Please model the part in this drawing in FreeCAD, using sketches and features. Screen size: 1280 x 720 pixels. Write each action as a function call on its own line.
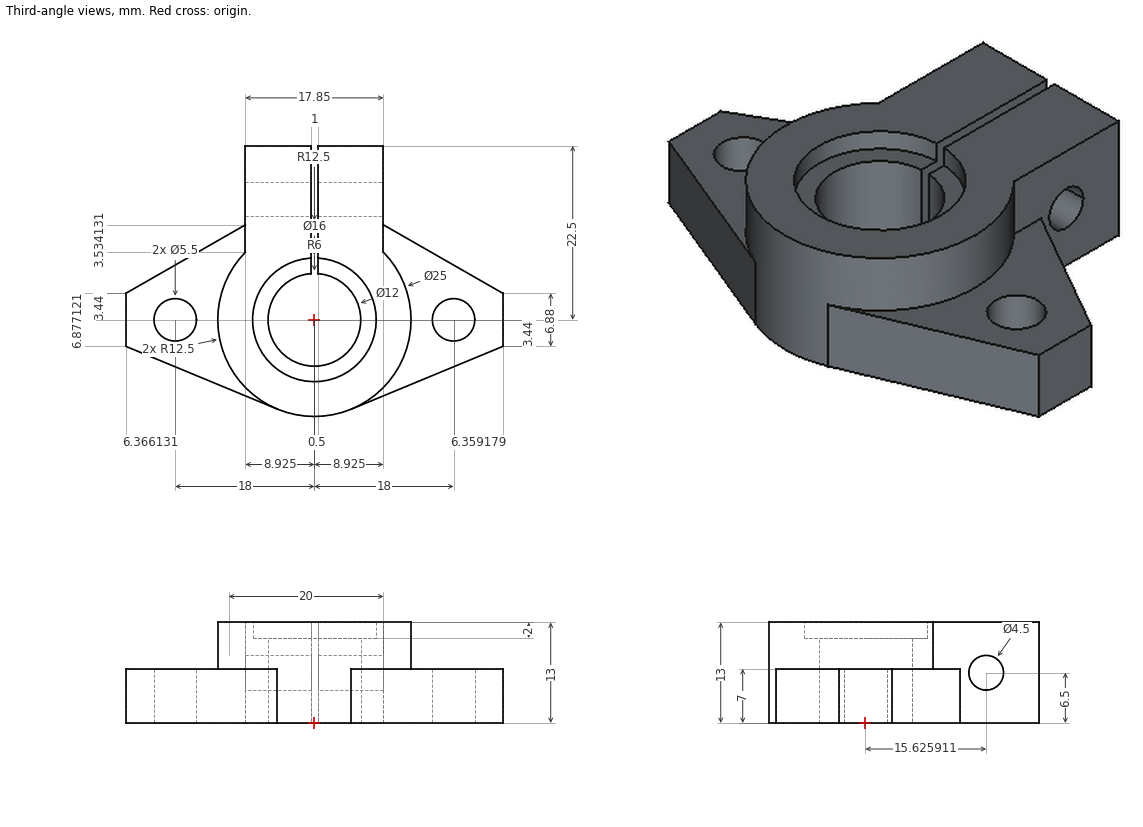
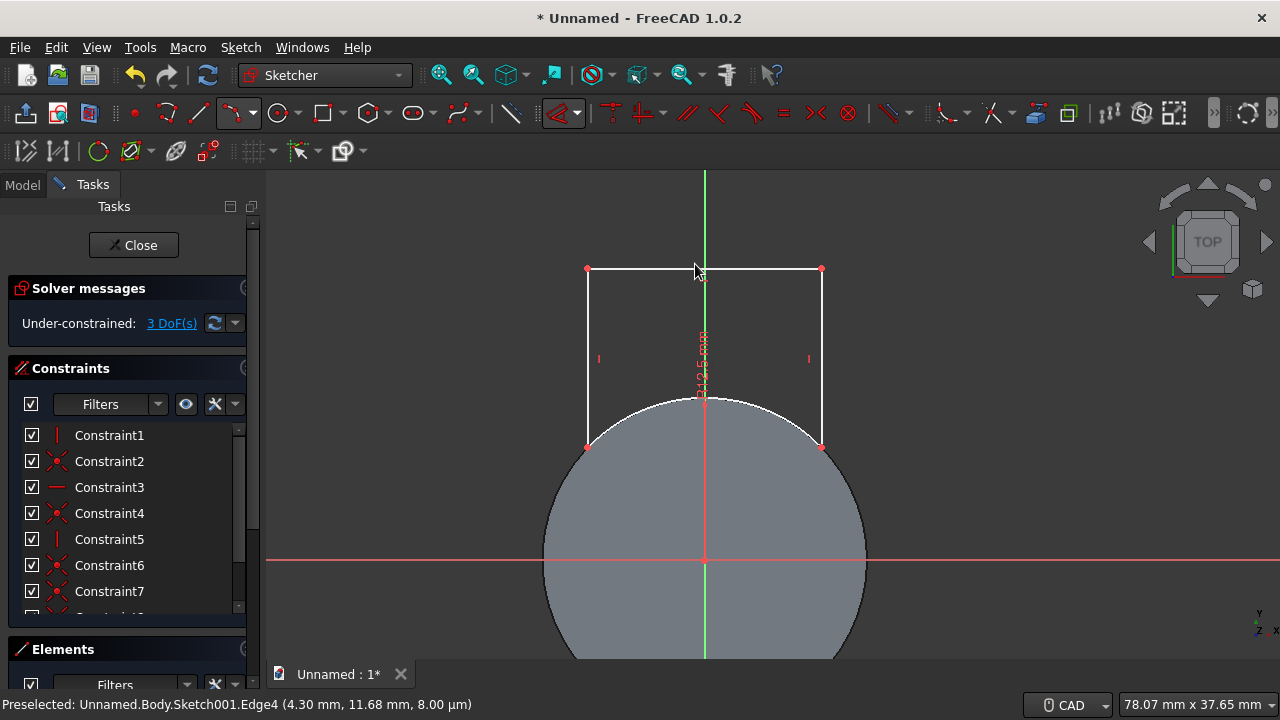
click(752, 269)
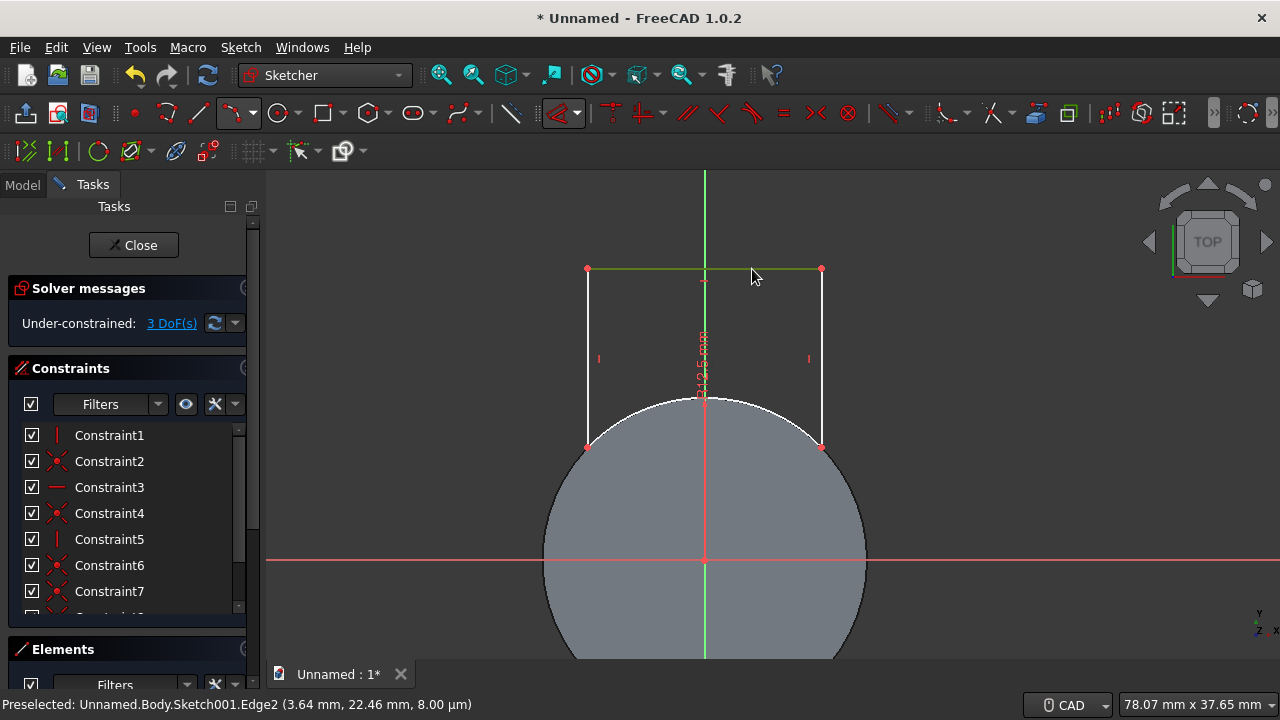
click(580, 114)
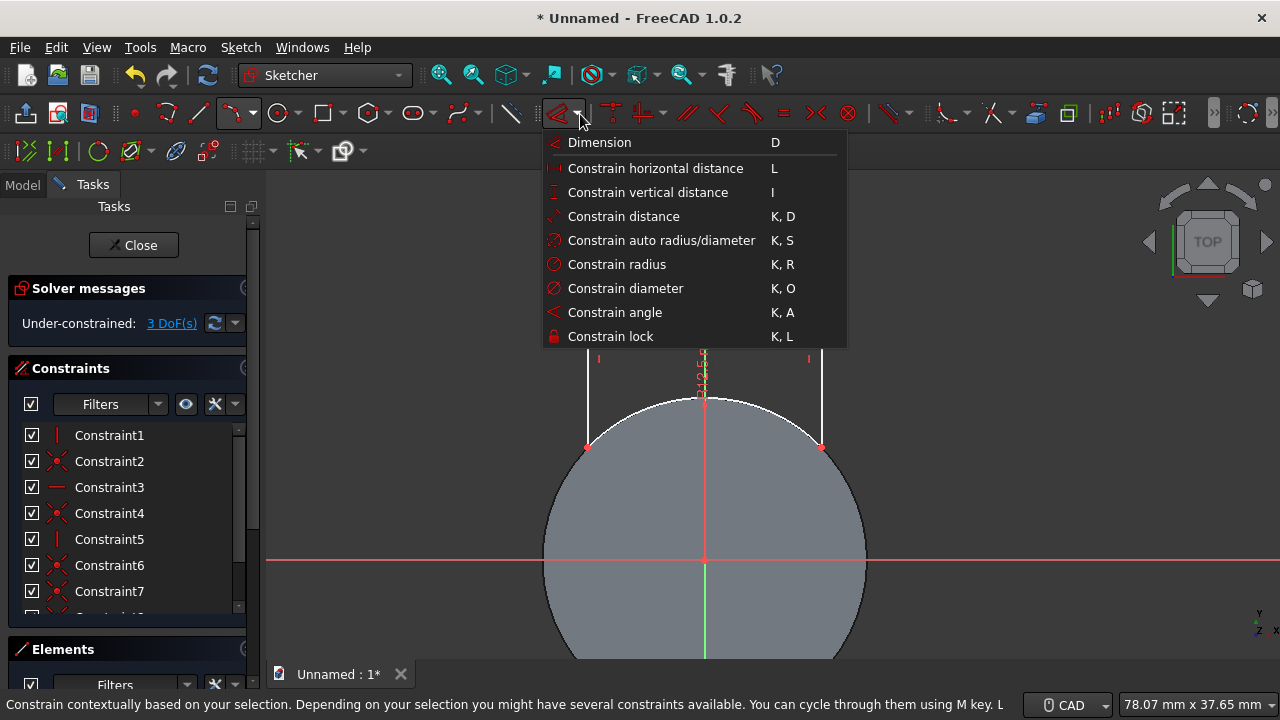
click(695, 168)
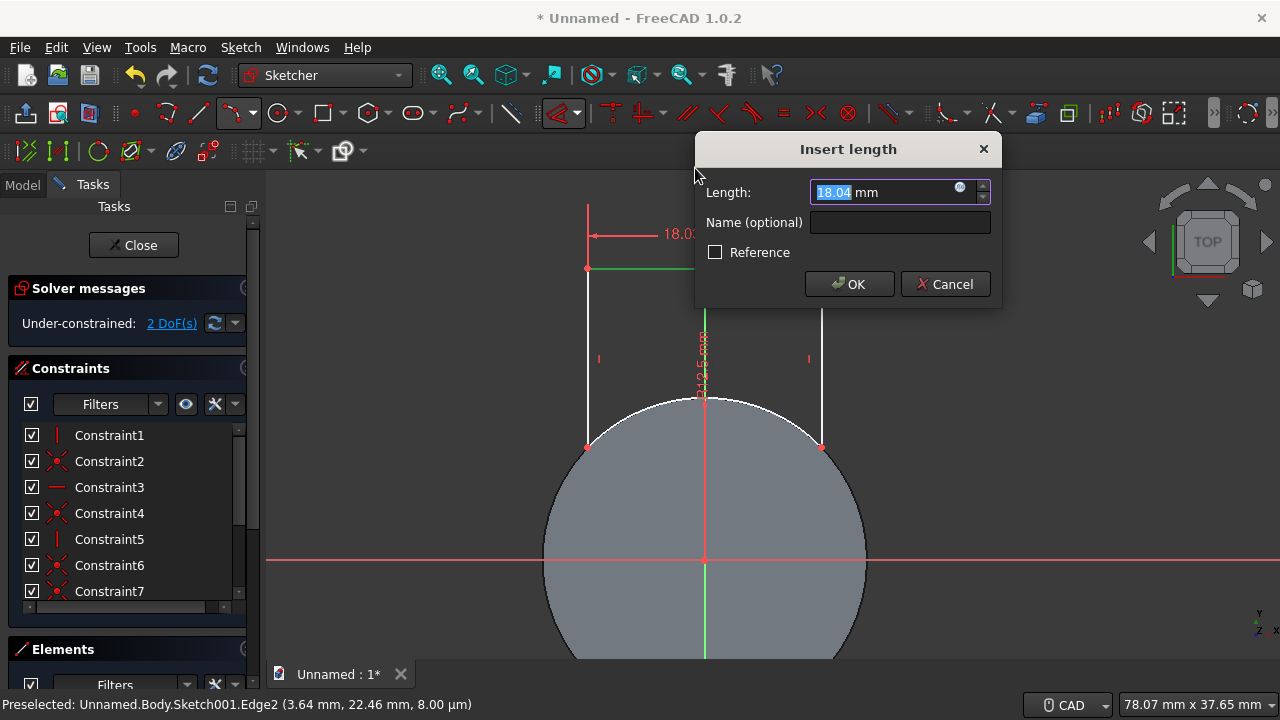
text(17.85)
key(Return)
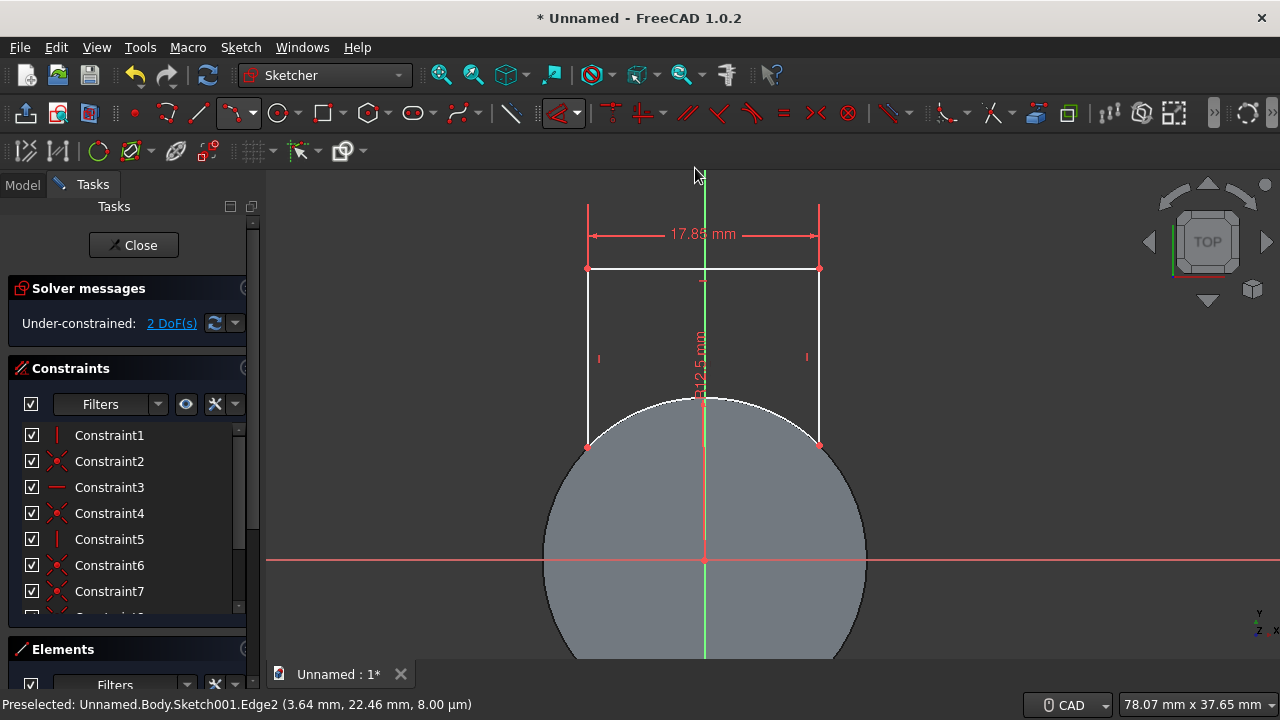
click(819, 269)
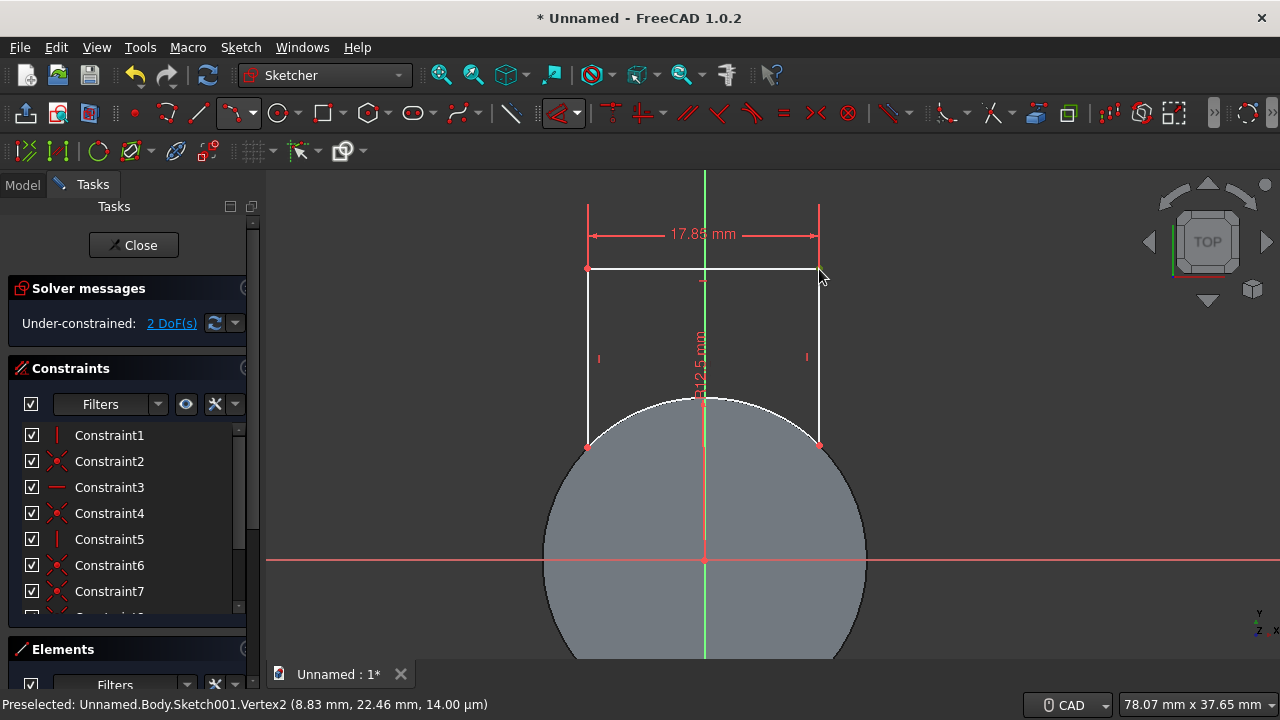
key(i)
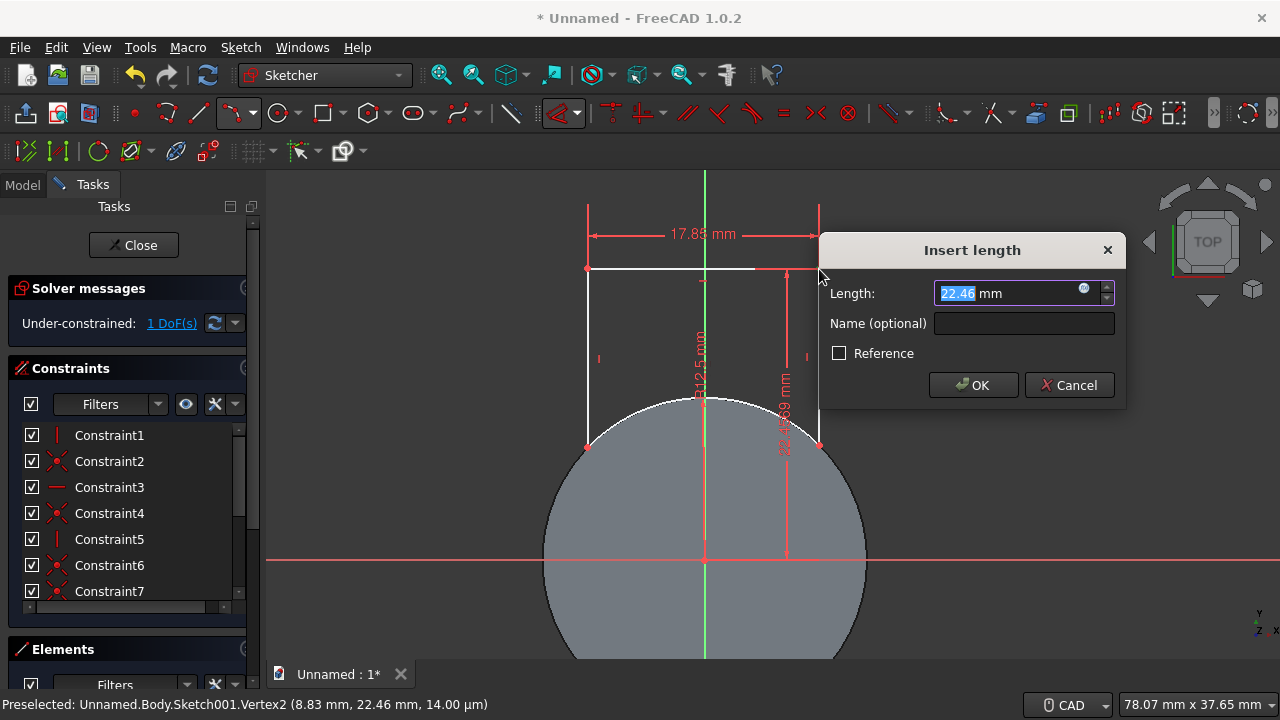
text(22.5)
key(Return)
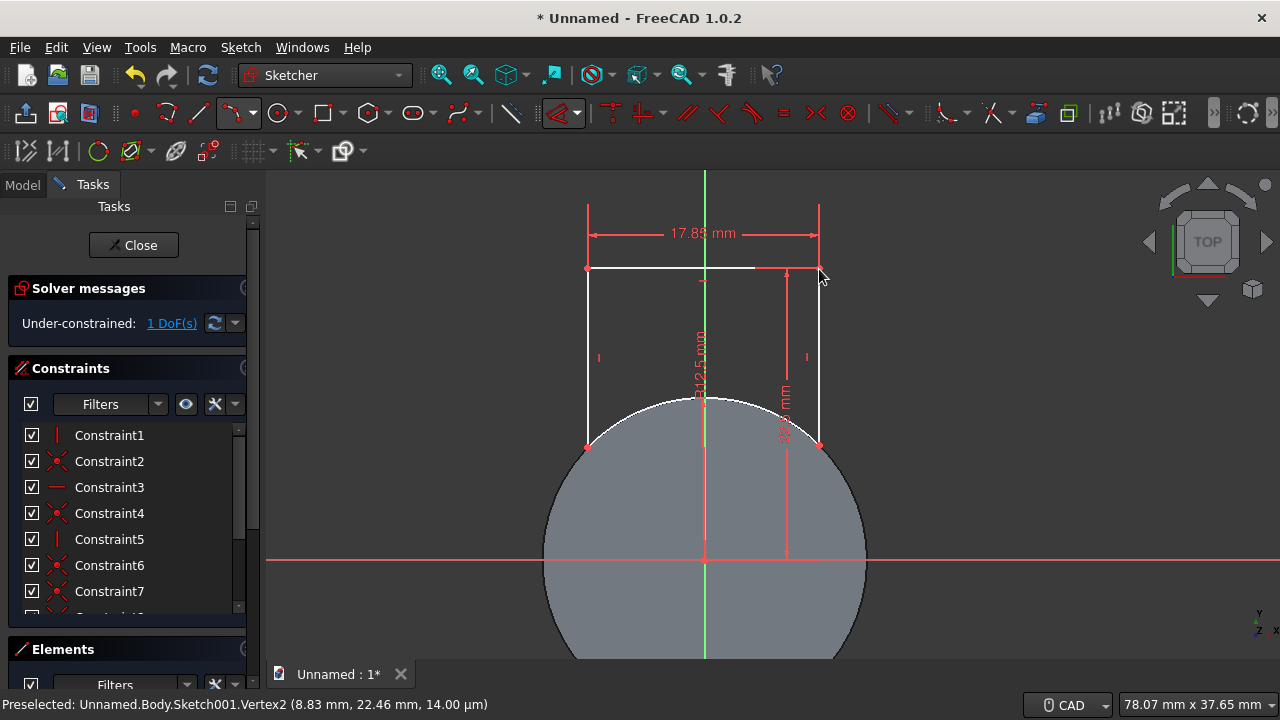
click(819, 445)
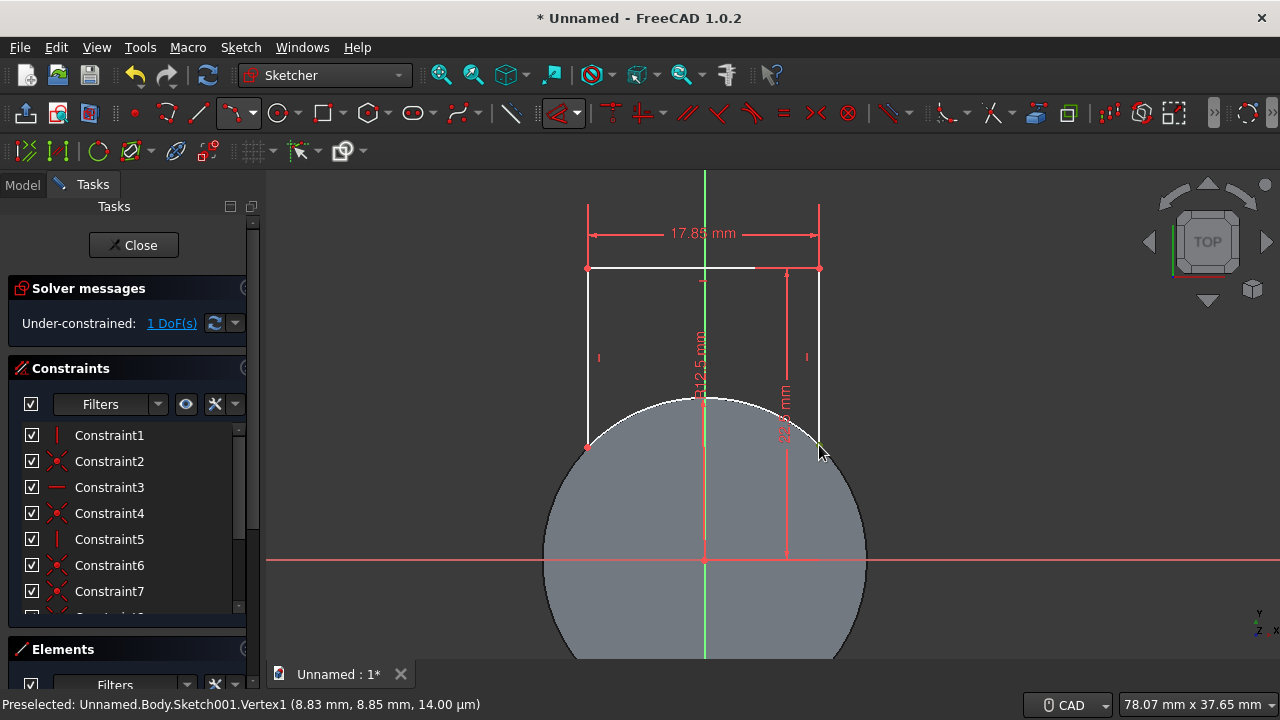
key(l)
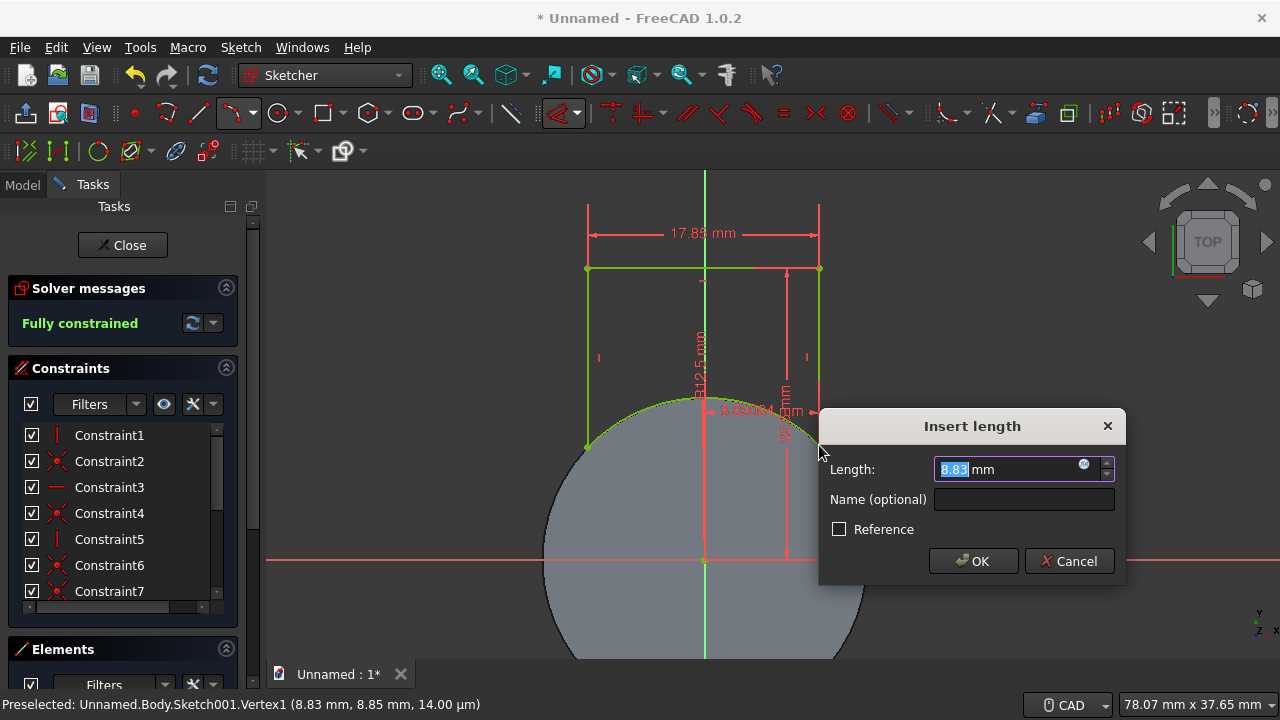
text(8.925)
key(Return)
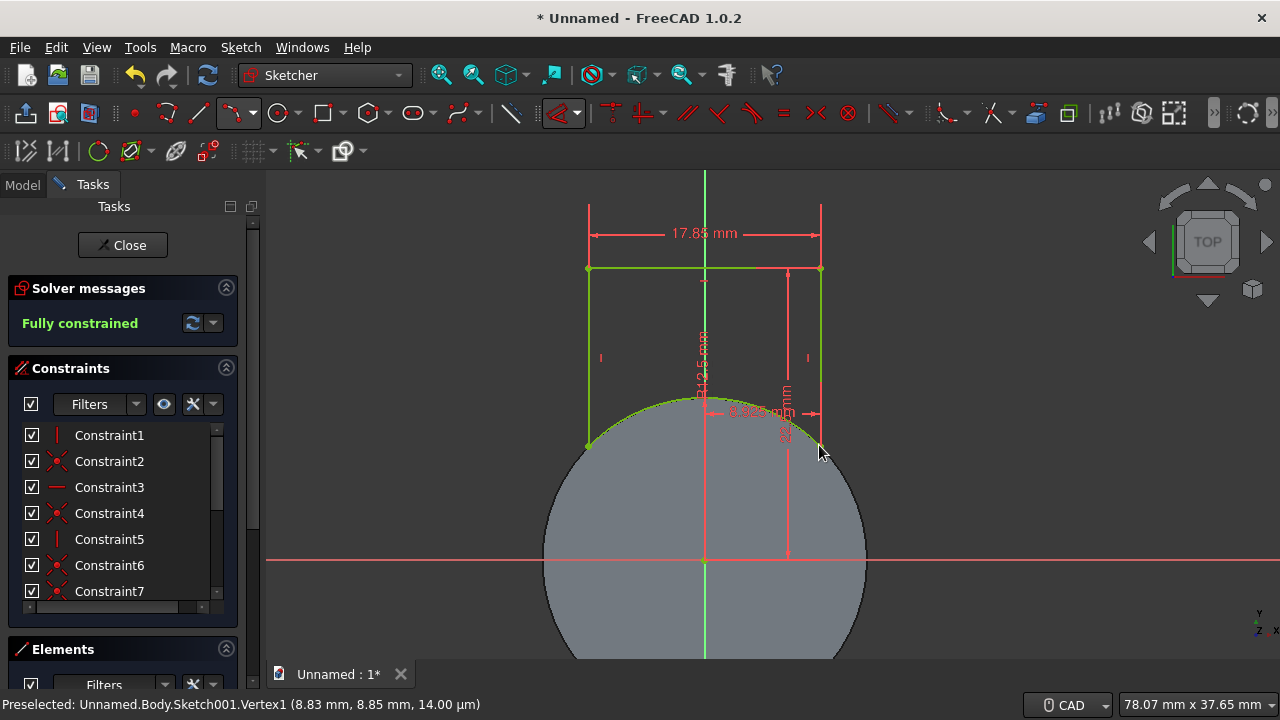
click(123, 245)